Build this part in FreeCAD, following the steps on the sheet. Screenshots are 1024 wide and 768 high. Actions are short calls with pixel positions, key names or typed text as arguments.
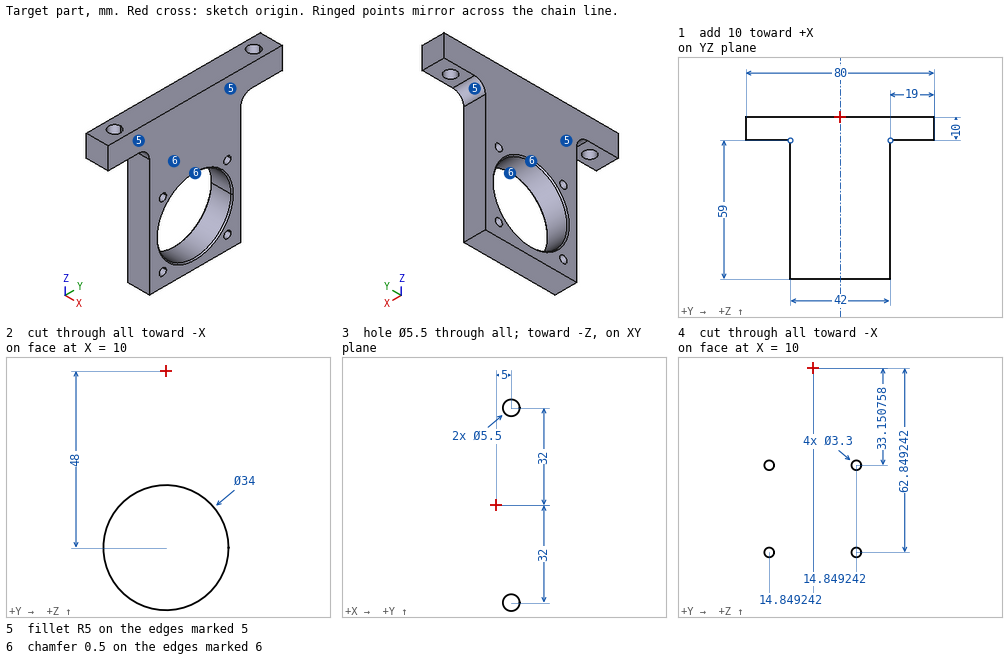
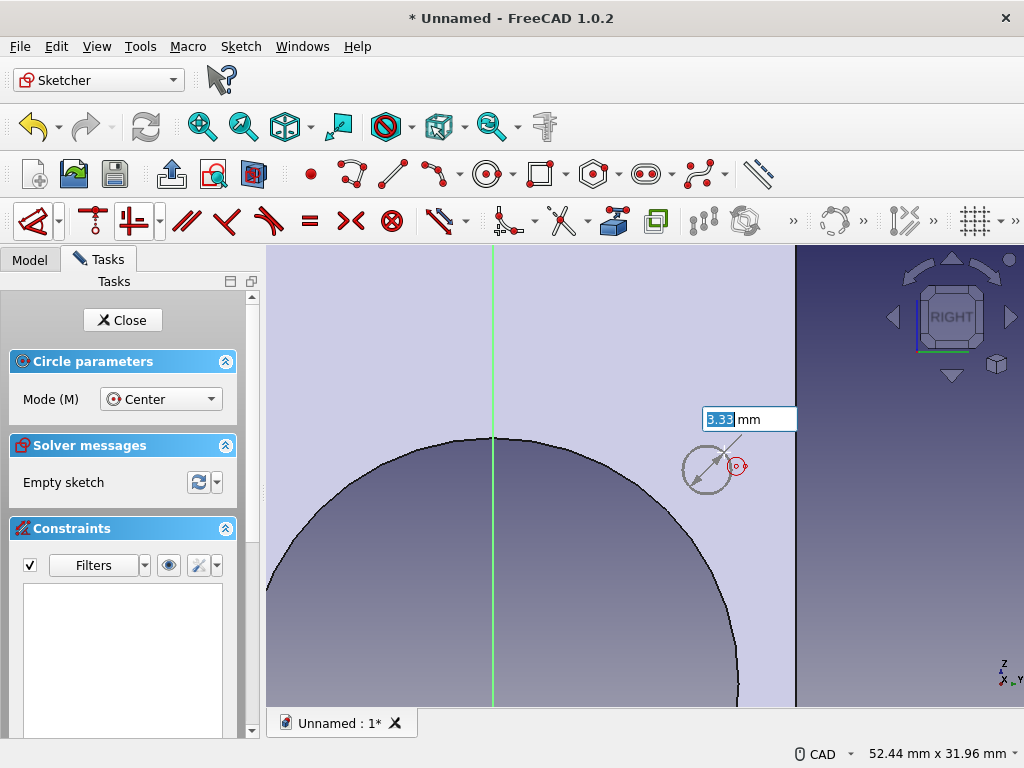
text(3.3)
key(Return)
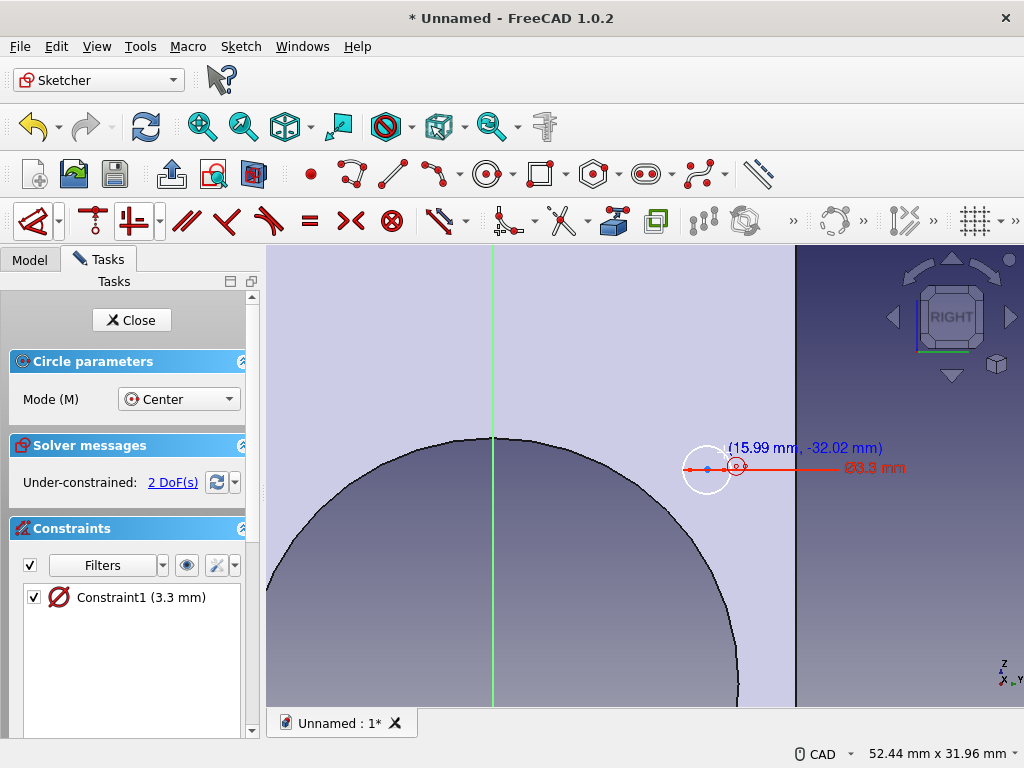
scroll(613, 485, down, 6)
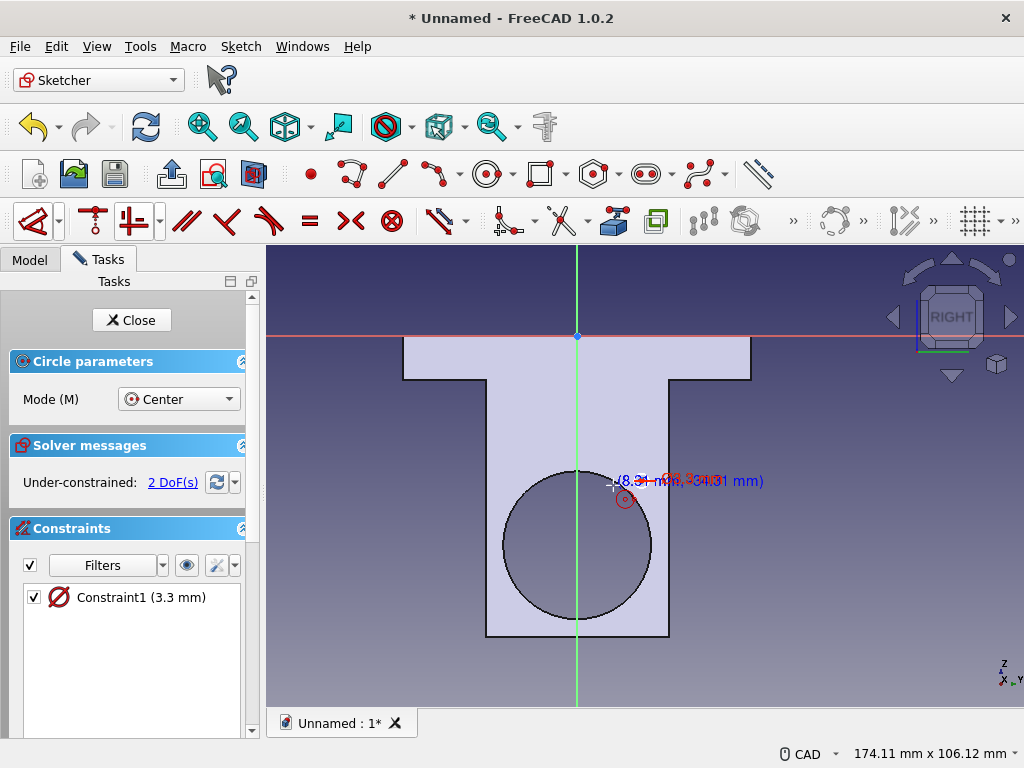
scroll(642, 610, up, 6)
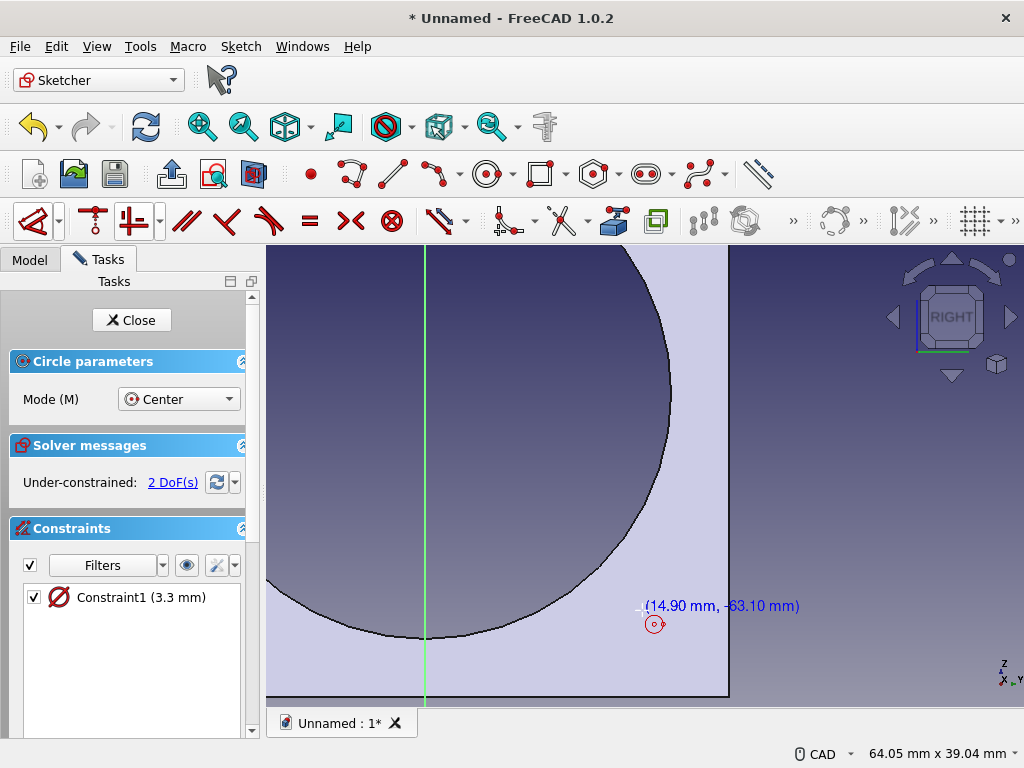
click(640, 608)
move(657, 591)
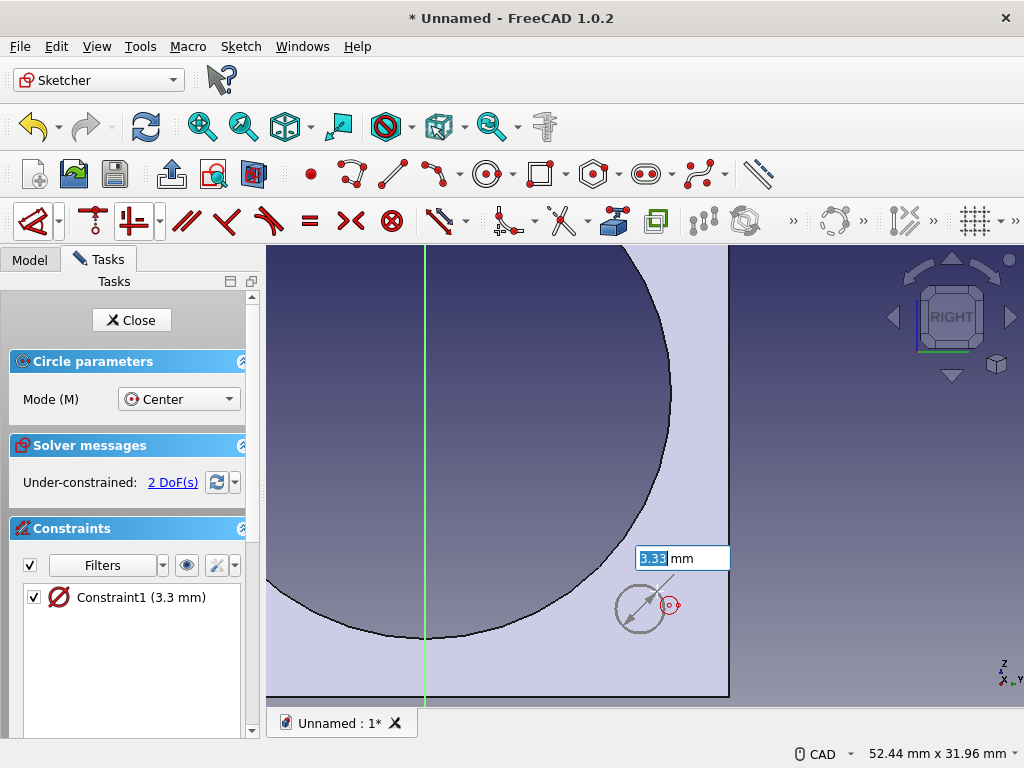
text(3.3)
key(Return)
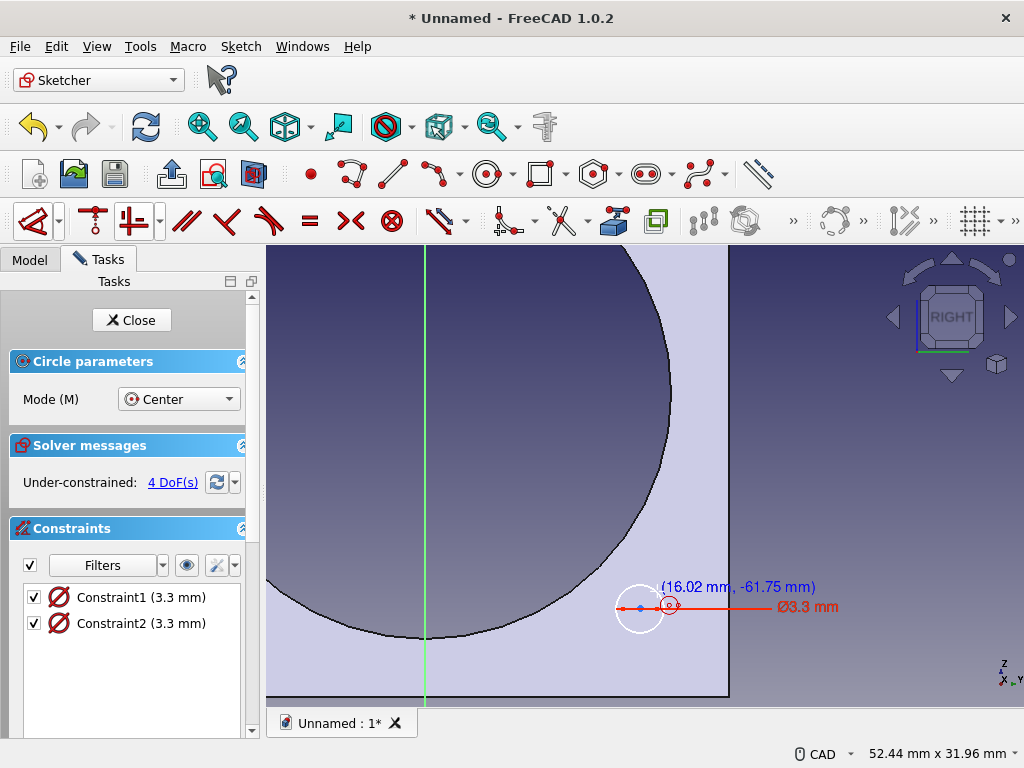
scroll(642, 610, down, 6)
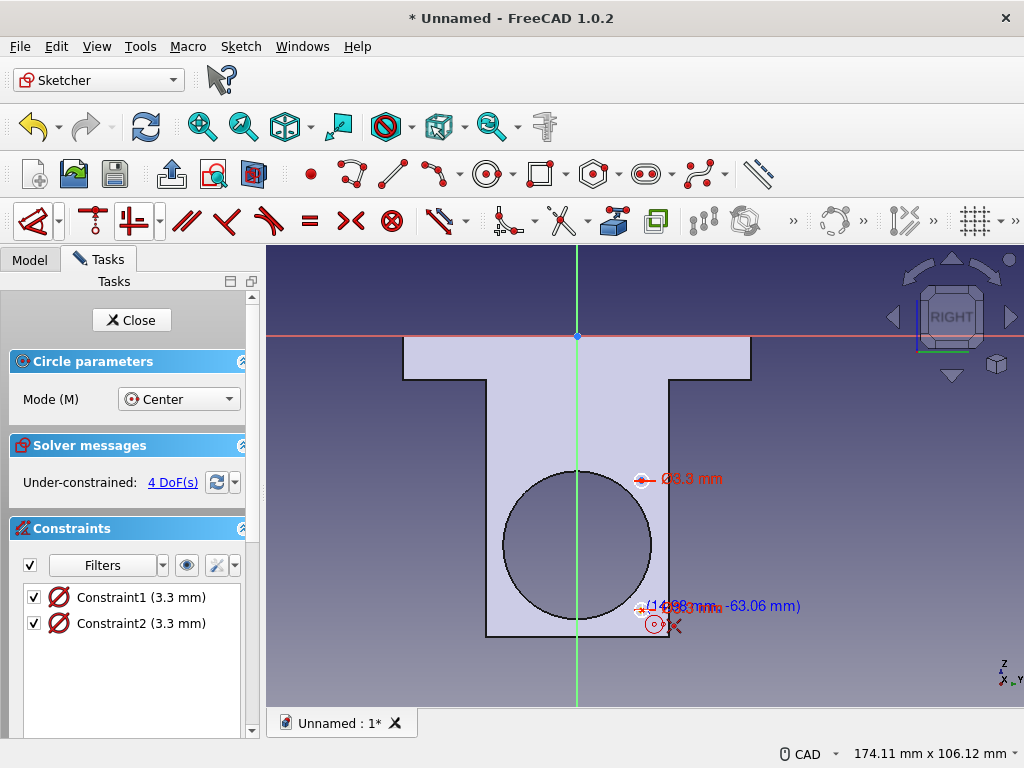
scroll(512, 610, up, 6)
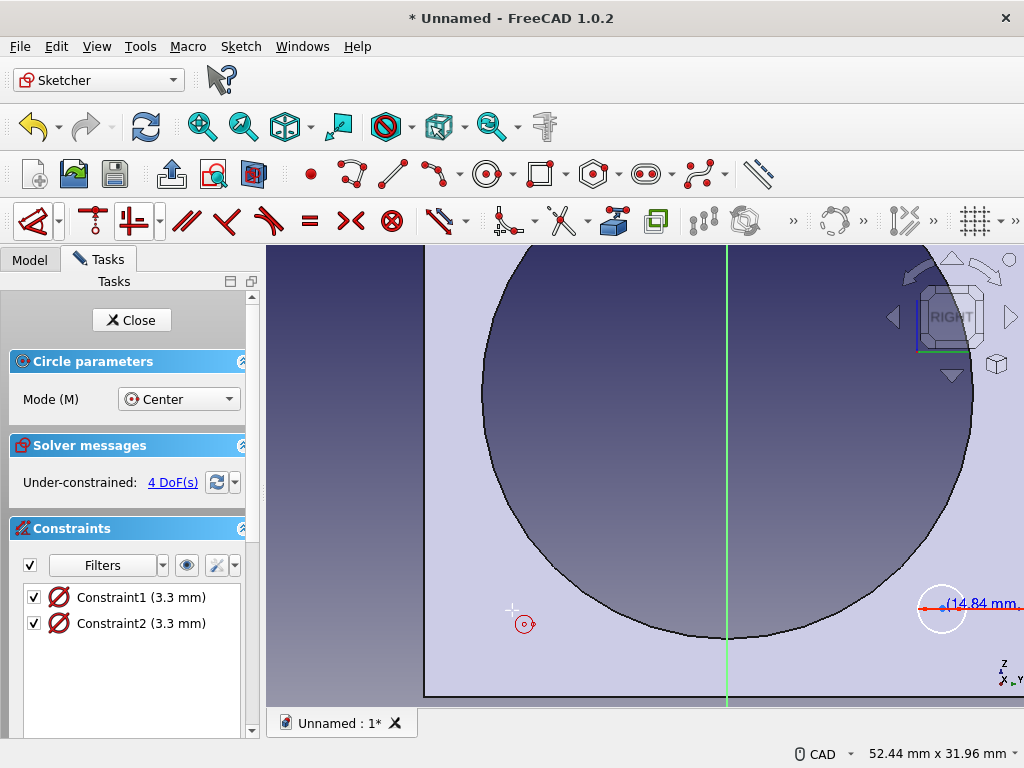
click(513, 608)
move(530, 591)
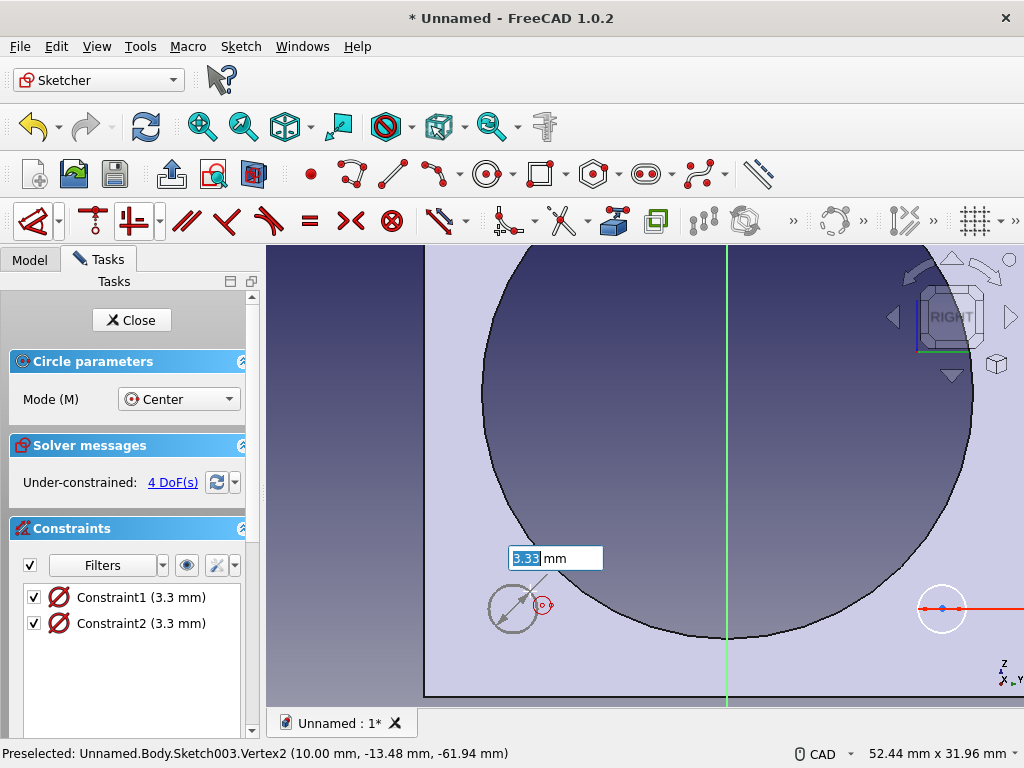
text(3.3)
key(Return)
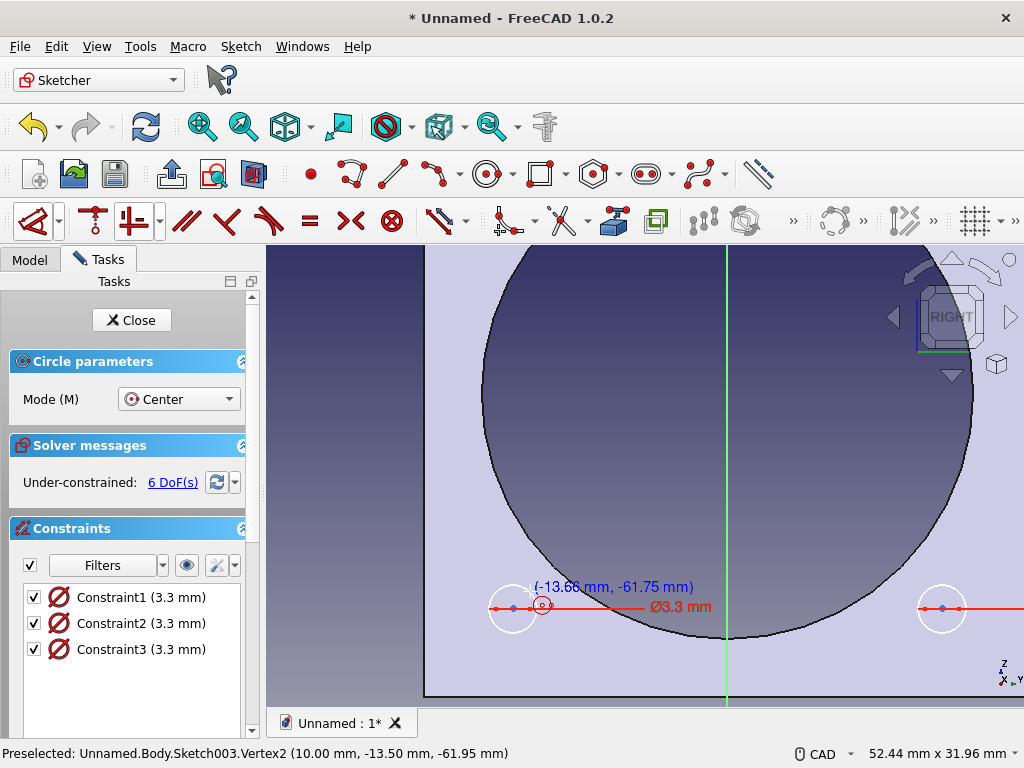
scroll(511, 610, down, 6)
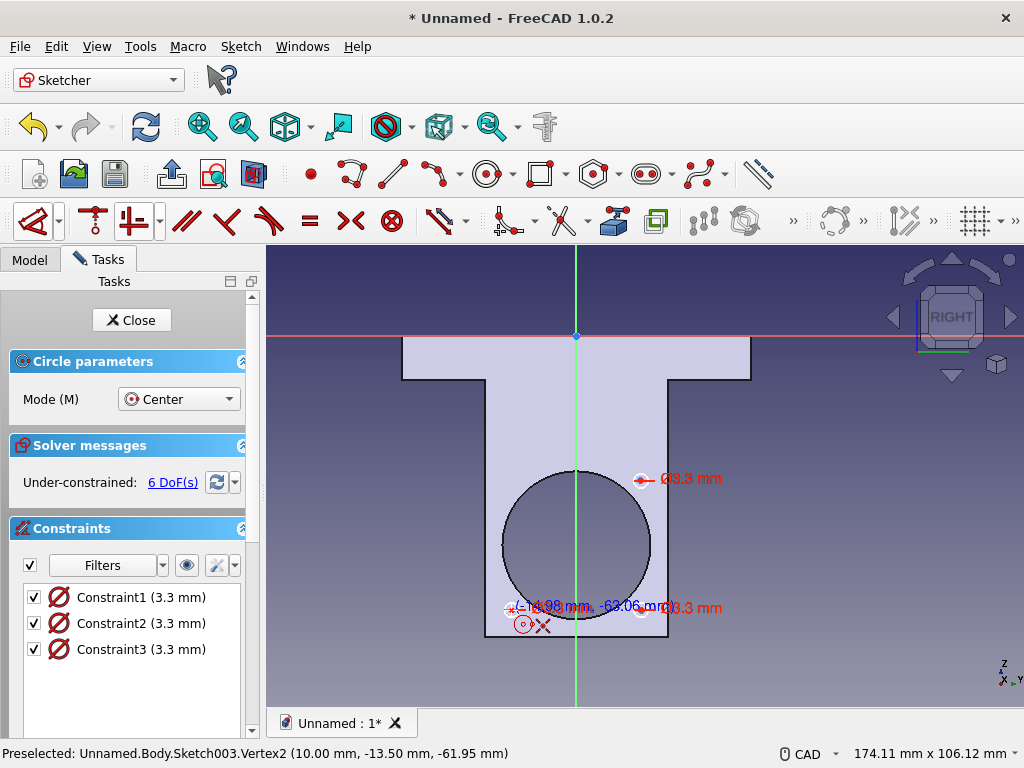
scroll(512, 481, up, 6)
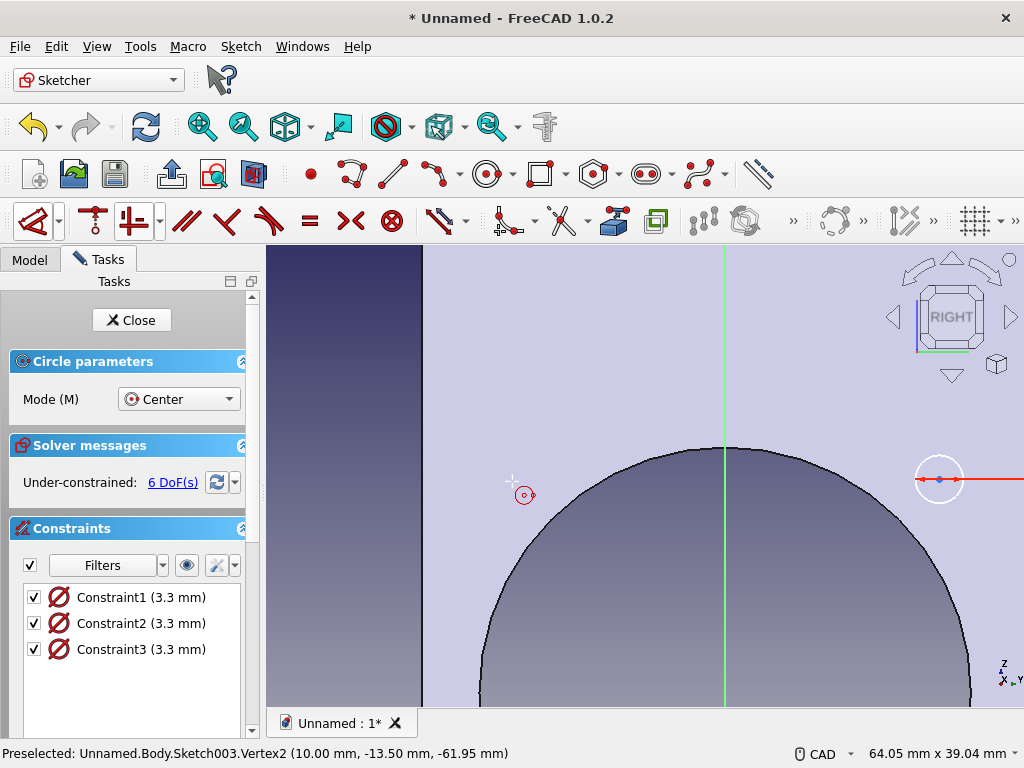
click(511, 479)
move(527, 462)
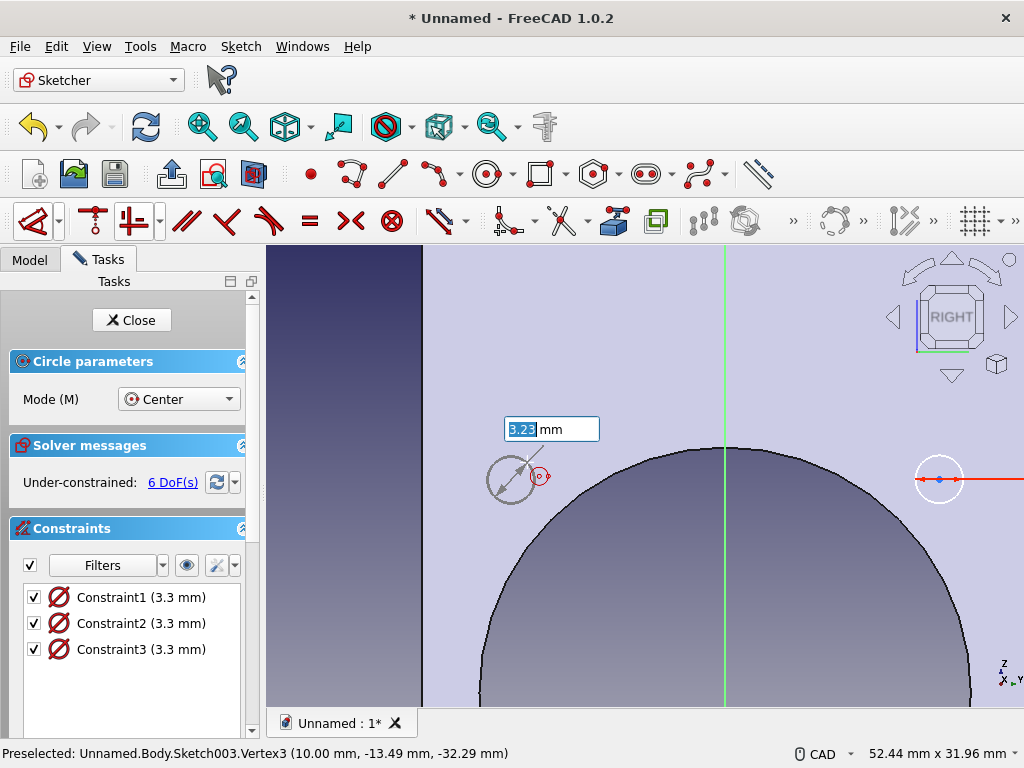
text(3.3)
key(Return)
key(Escape)